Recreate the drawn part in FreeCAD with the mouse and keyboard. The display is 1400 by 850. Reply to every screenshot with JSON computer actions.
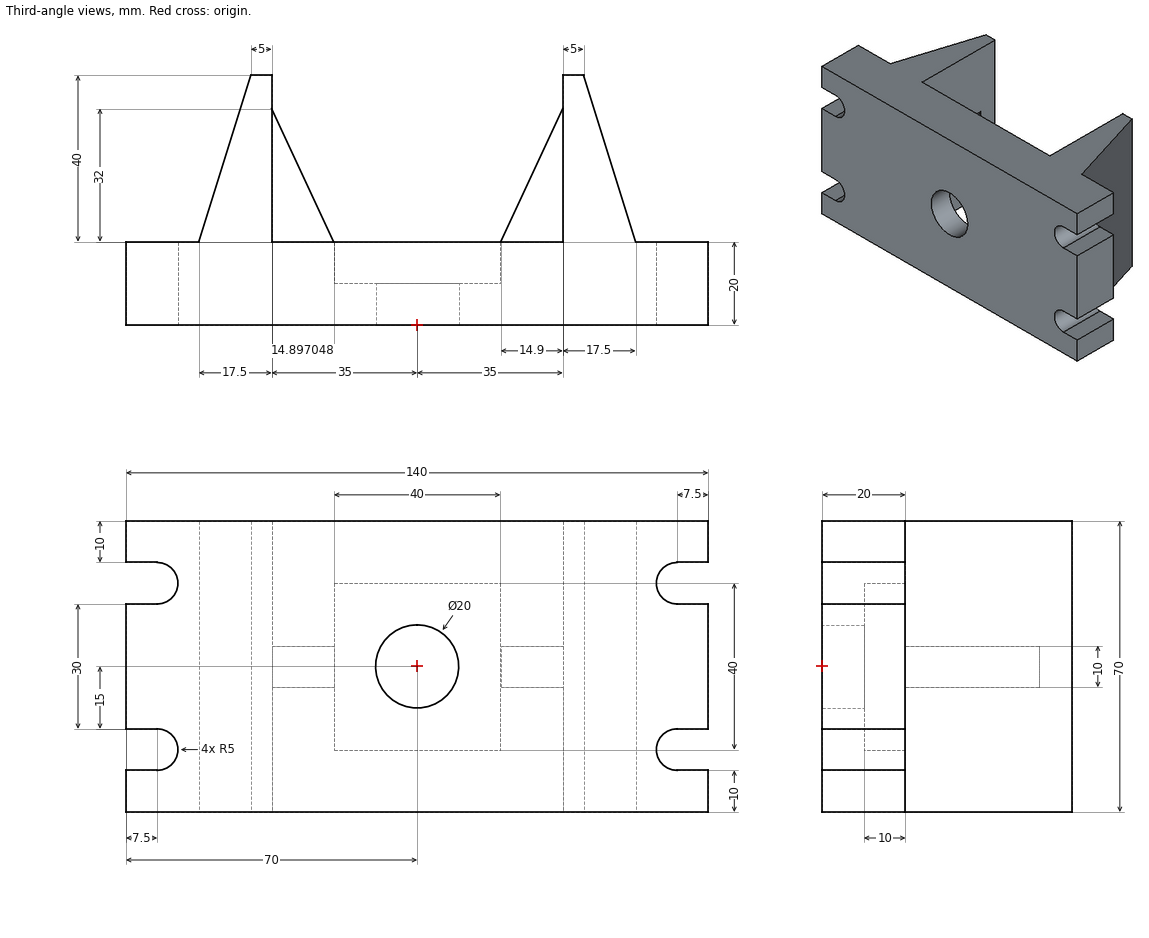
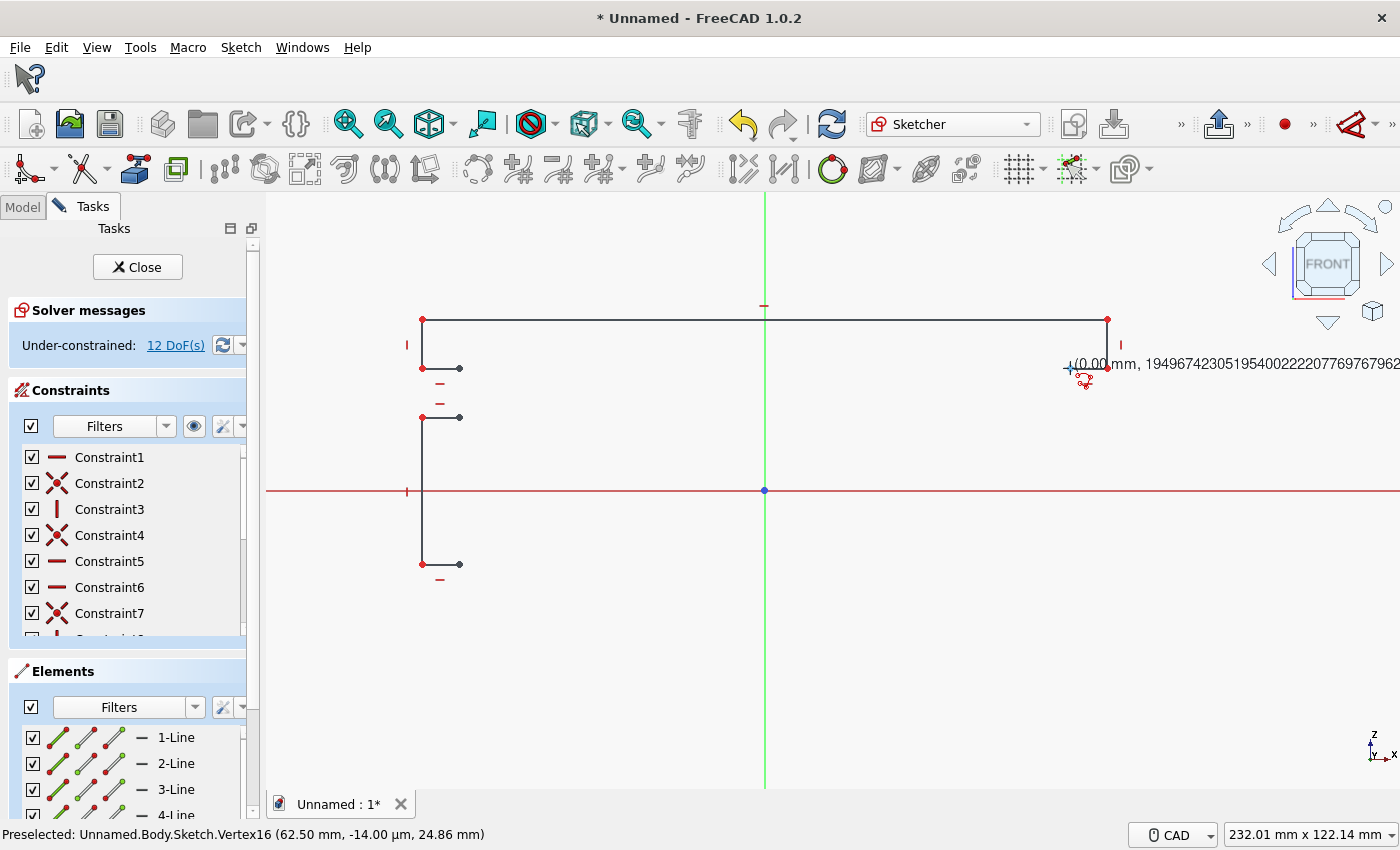
{"action": "left_click", "coordinate": [1070, 417]}
{"action": "left_click", "coordinate": [1107, 417]}
{"action": "left_click", "coordinate": [1107, 564]}
{"action": "left_click", "coordinate": [1070, 564]}
{"action": "right_click", "coordinate": [1070, 564]}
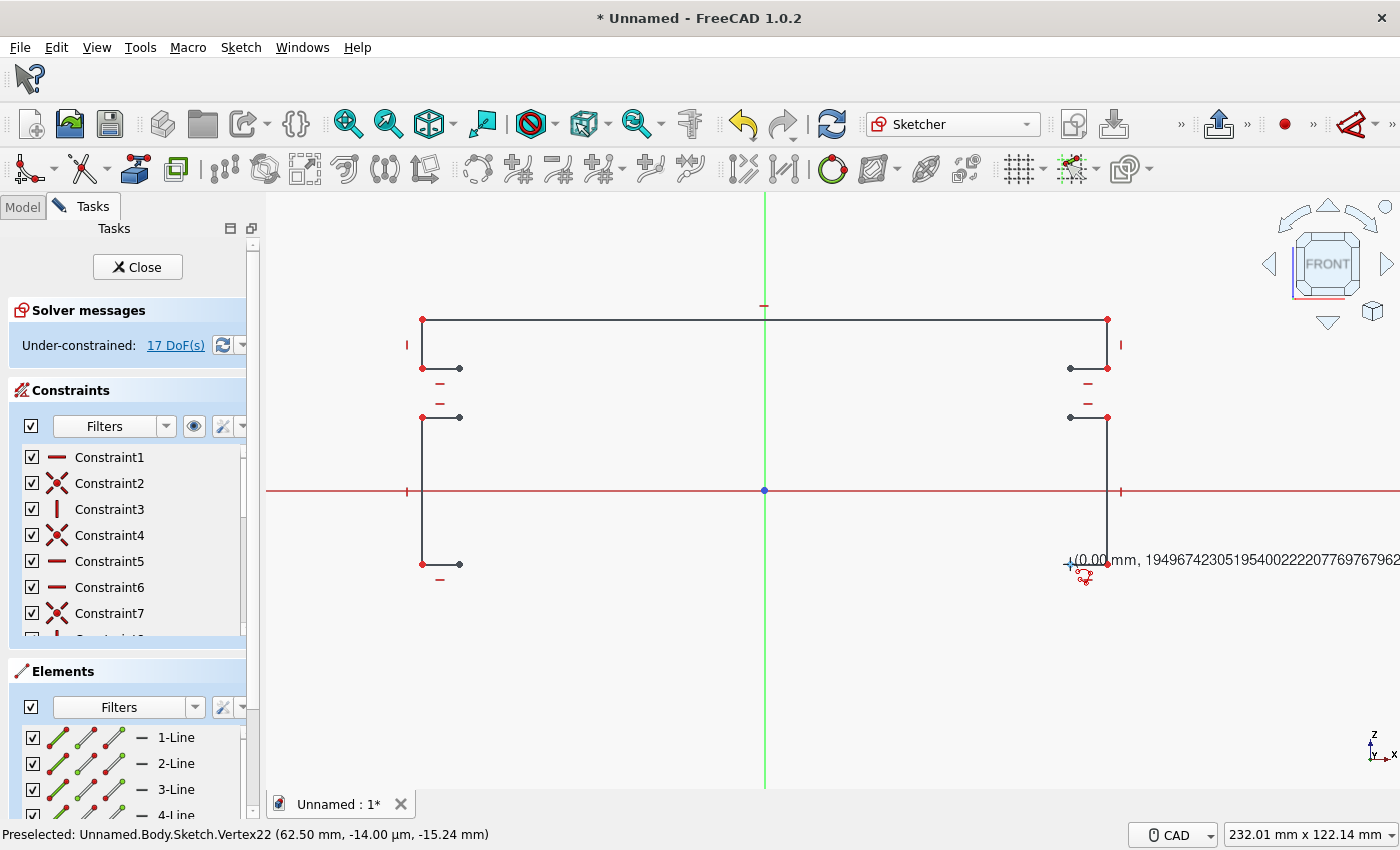
{"action": "left_click", "coordinate": [1070, 613]}
{"action": "left_click", "coordinate": [1107, 613]}
{"action": "left_click", "coordinate": [1107, 662]}
{"action": "left_click", "coordinate": [422, 662]}
{"action": "left_click", "coordinate": [422, 613]}
{"action": "left_click", "coordinate": [459, 613]}
{"action": "right_click", "coordinate": [459, 613]}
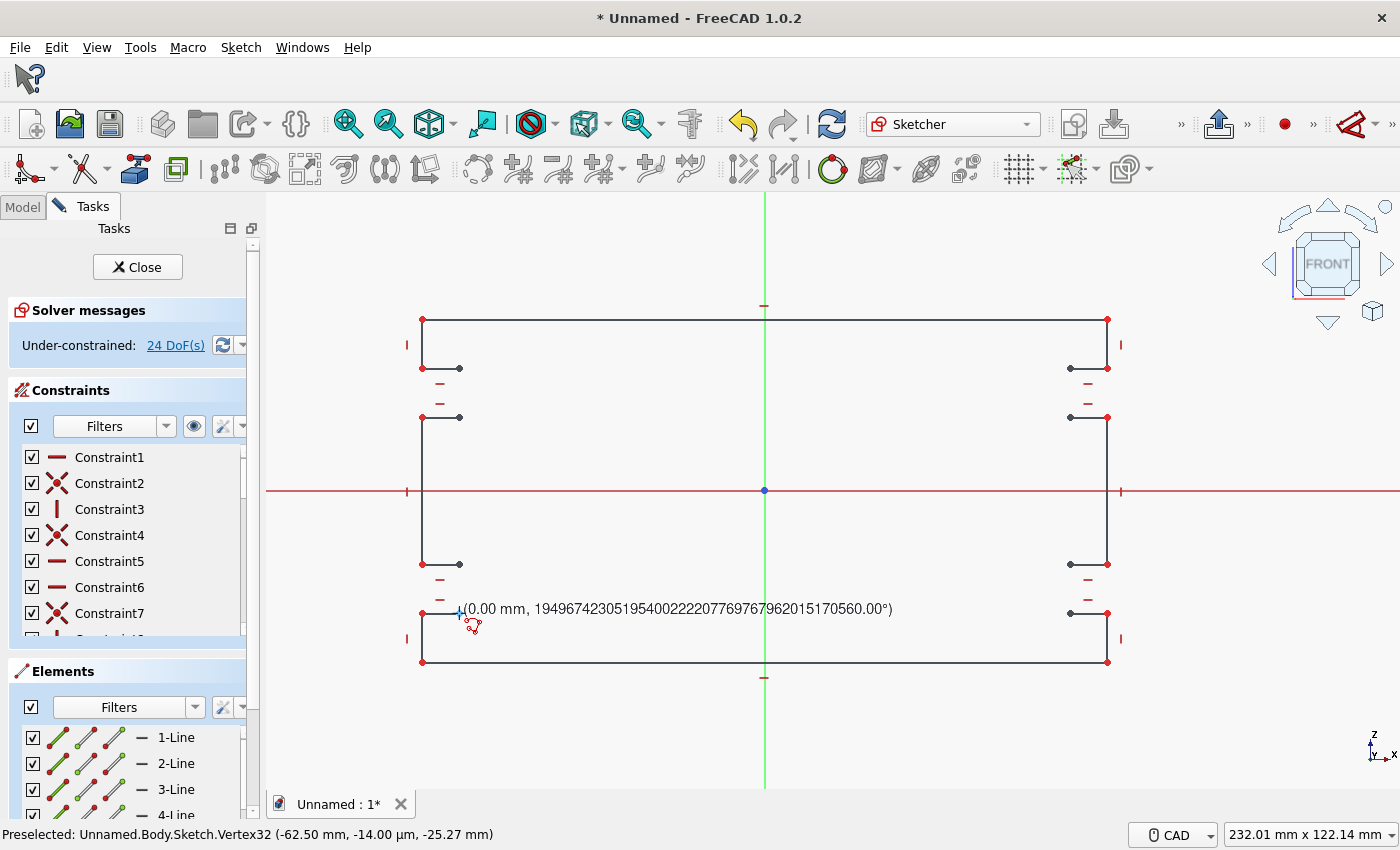
{"action": "key", "text": "g 3 a"}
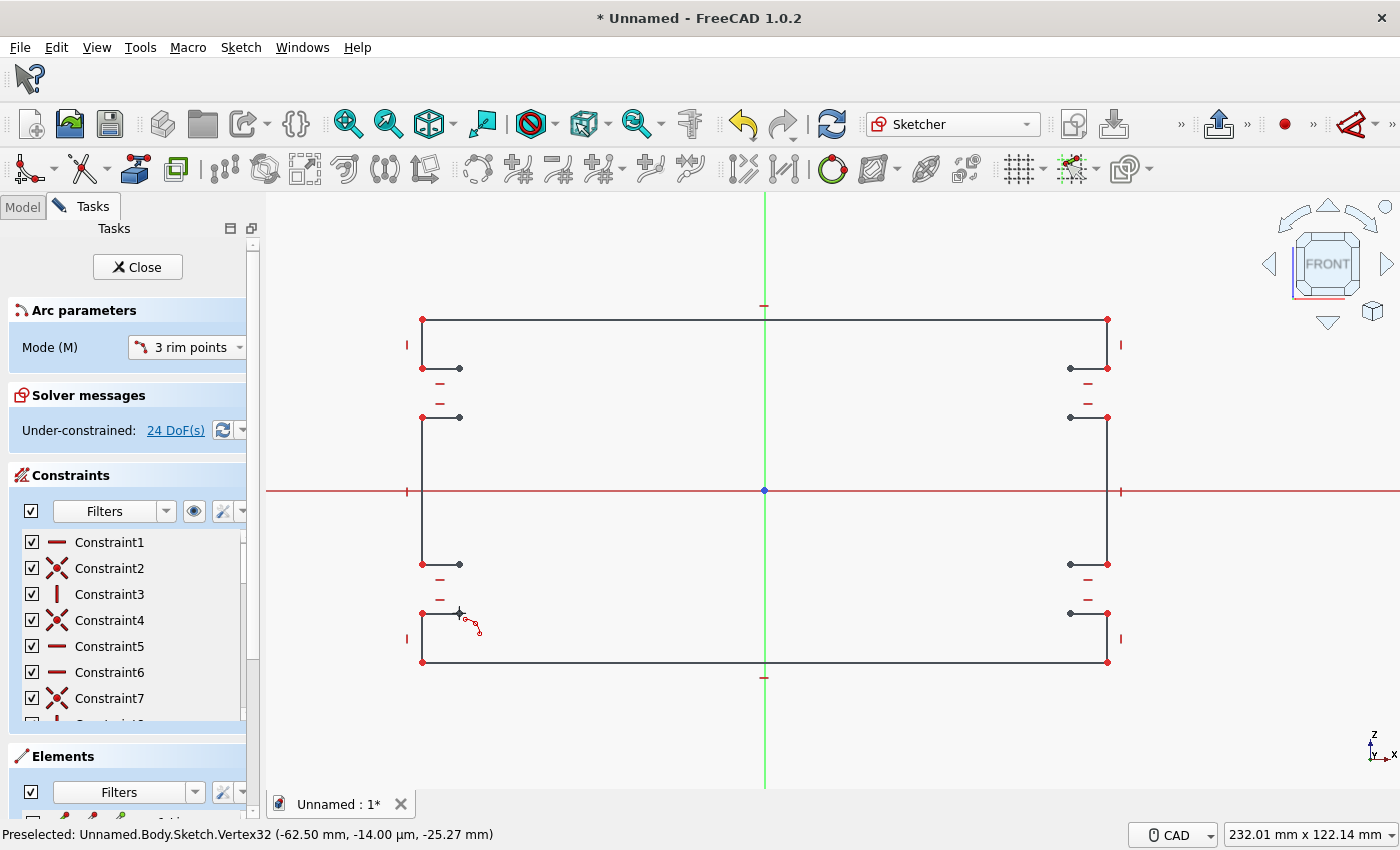
{"action": "left_click", "coordinate": [459, 418]}
{"action": "left_click", "coordinate": [459, 369]}
{"action": "left_click", "coordinate": [483, 393]}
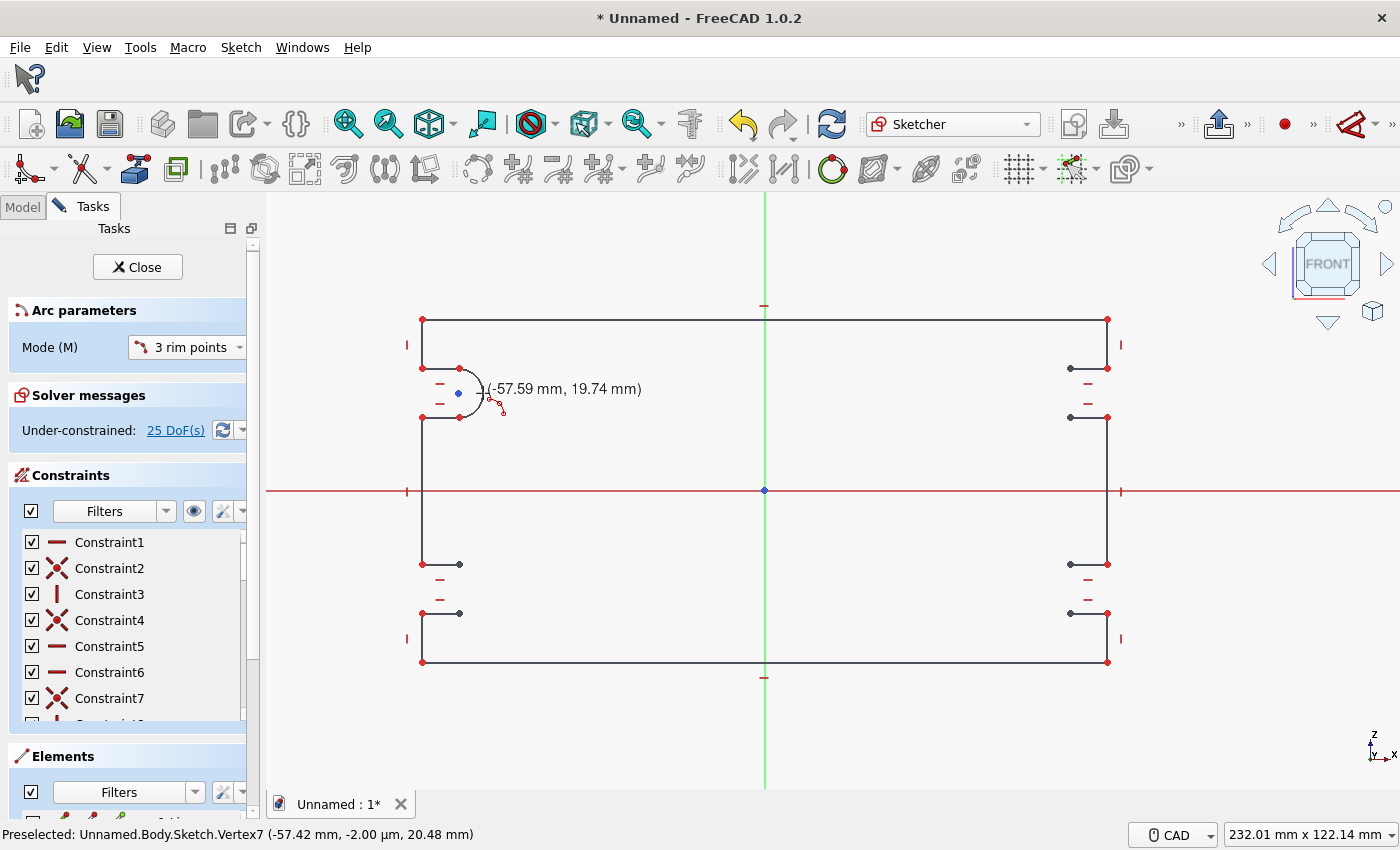
{"action": "left_click", "coordinate": [1070, 369]}
{"action": "left_click", "coordinate": [1070, 418]}
{"action": "left_click", "coordinate": [1046, 393]}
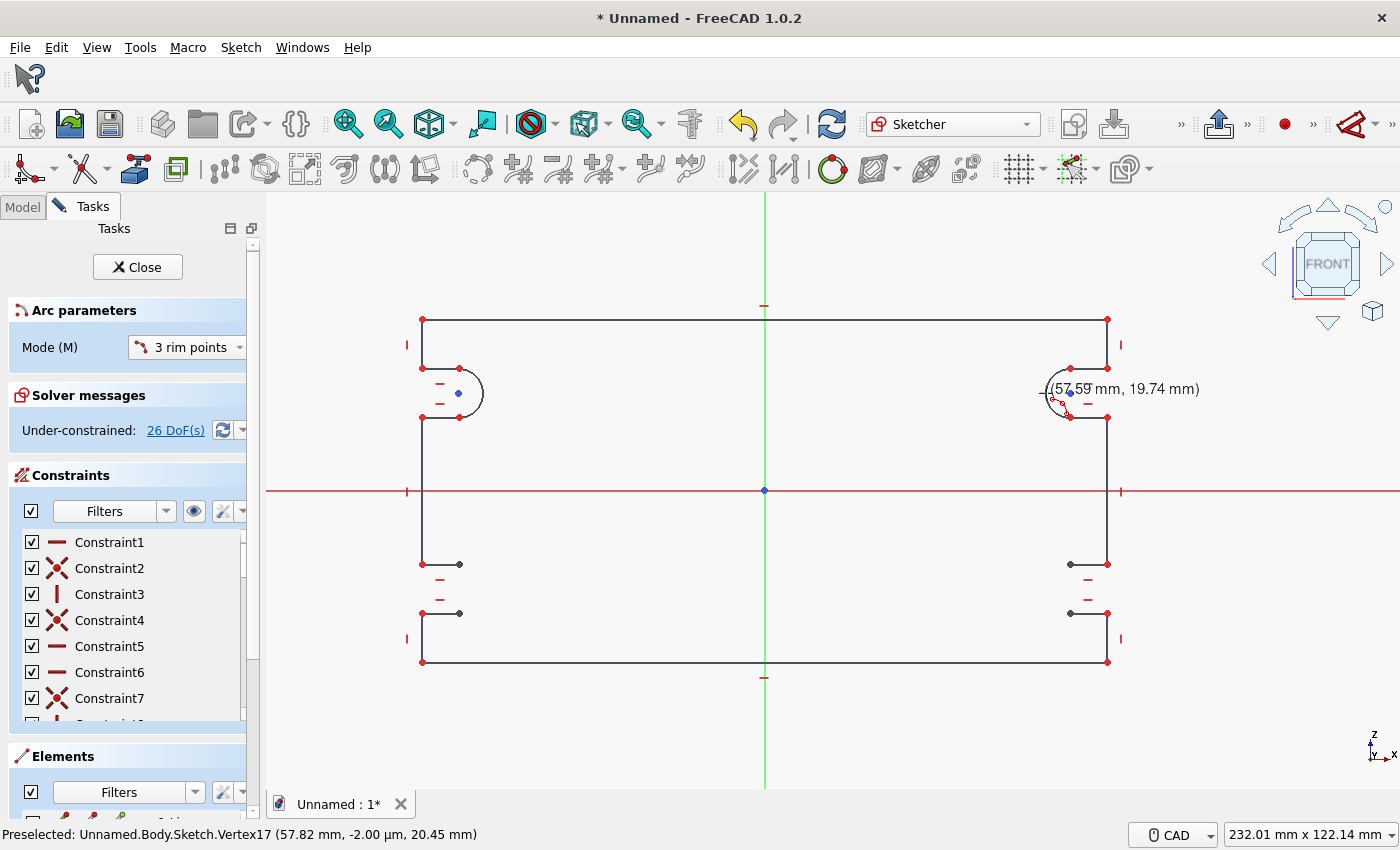
{"action": "left_click", "coordinate": [1070, 565]}
{"action": "left_click", "coordinate": [1070, 614]}
{"action": "left_click", "coordinate": [1046, 588]}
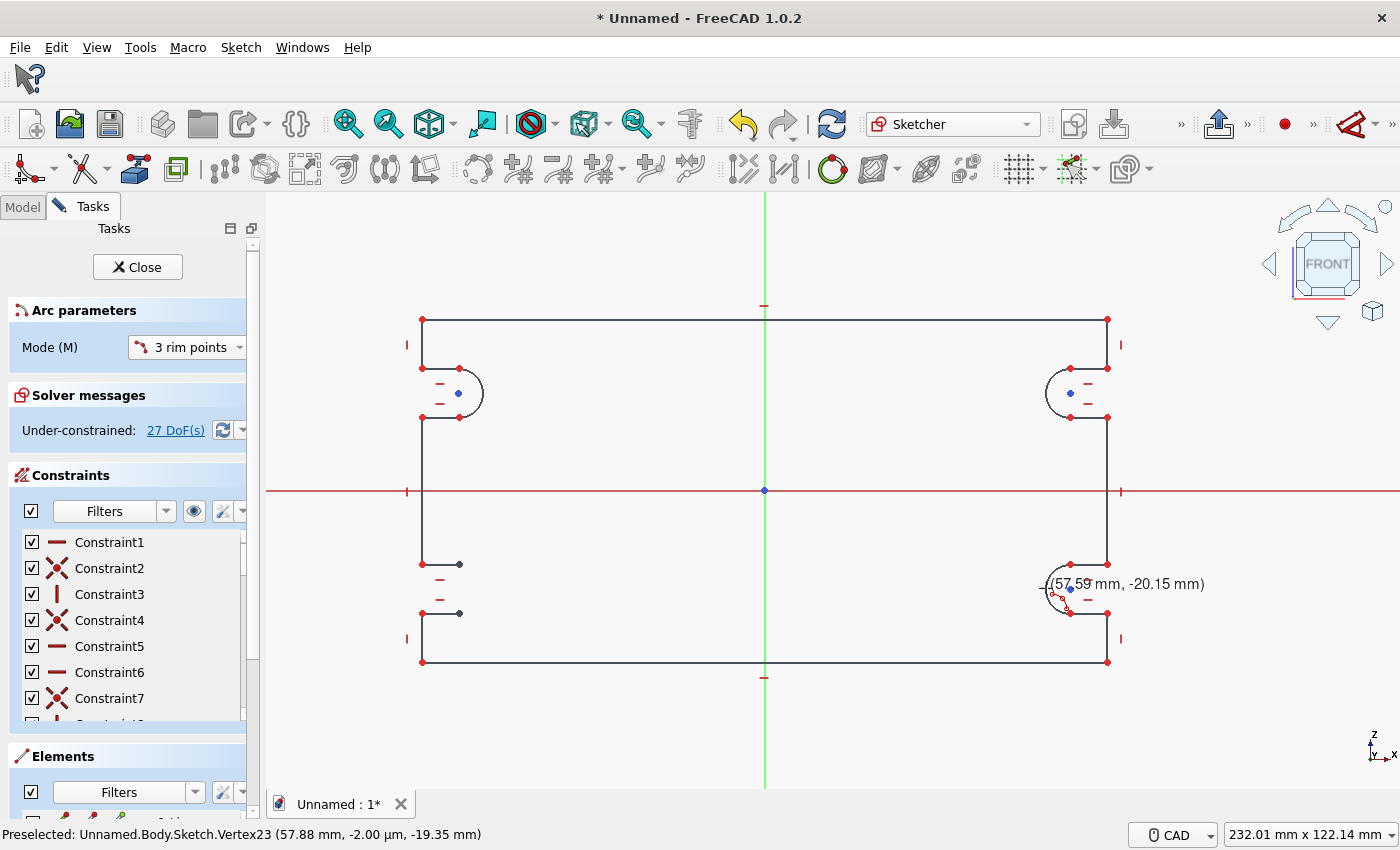
{"action": "left_click", "coordinate": [459, 614]}
{"action": "left_click", "coordinate": [459, 565]}
{"action": "left_click", "coordinate": [483, 588]}
{"action": "key", "text": "Escape"}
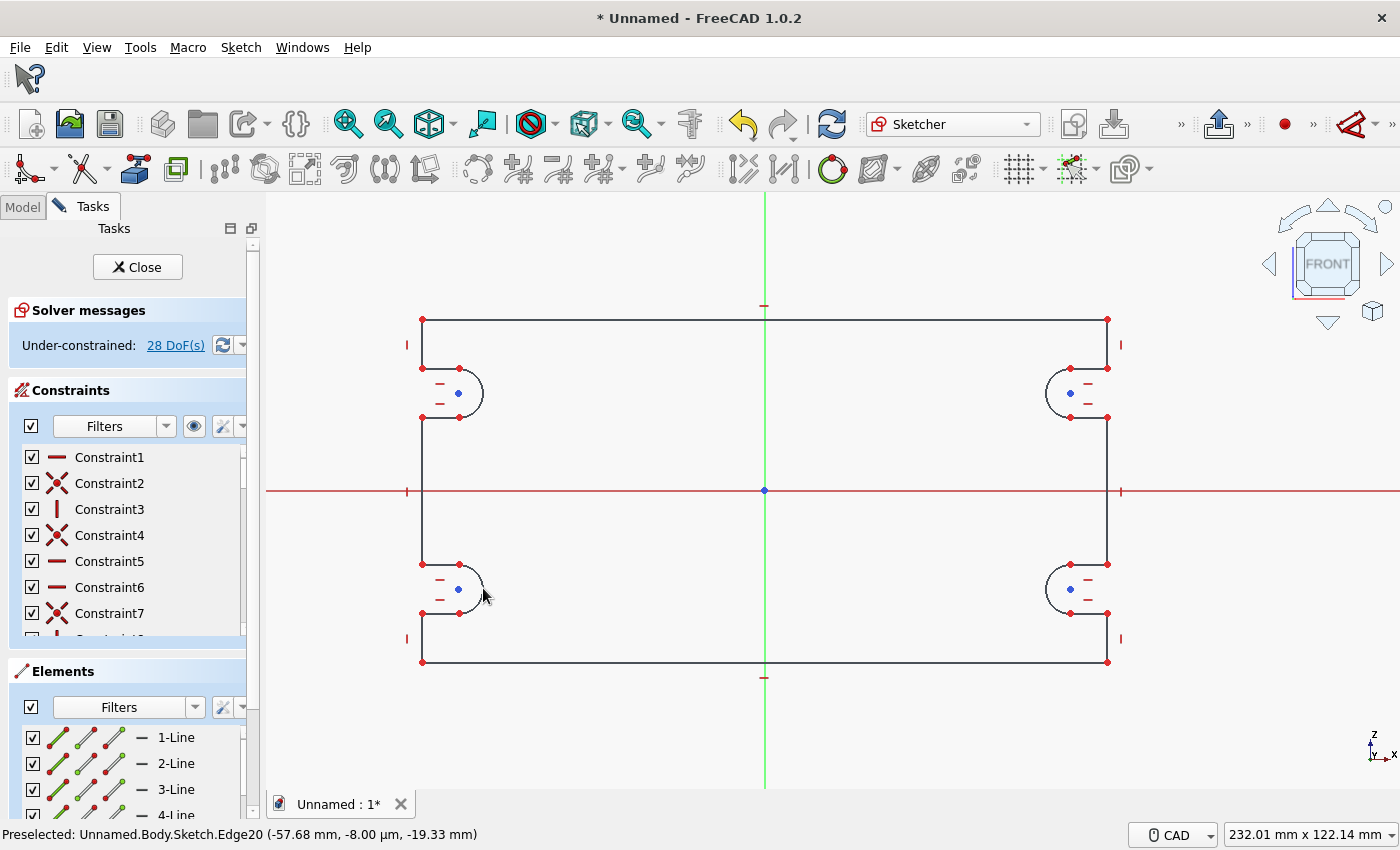
{"action": "scroll", "coordinate": [448, 565], "scroll_direction": "up", "scroll_amount": 2}